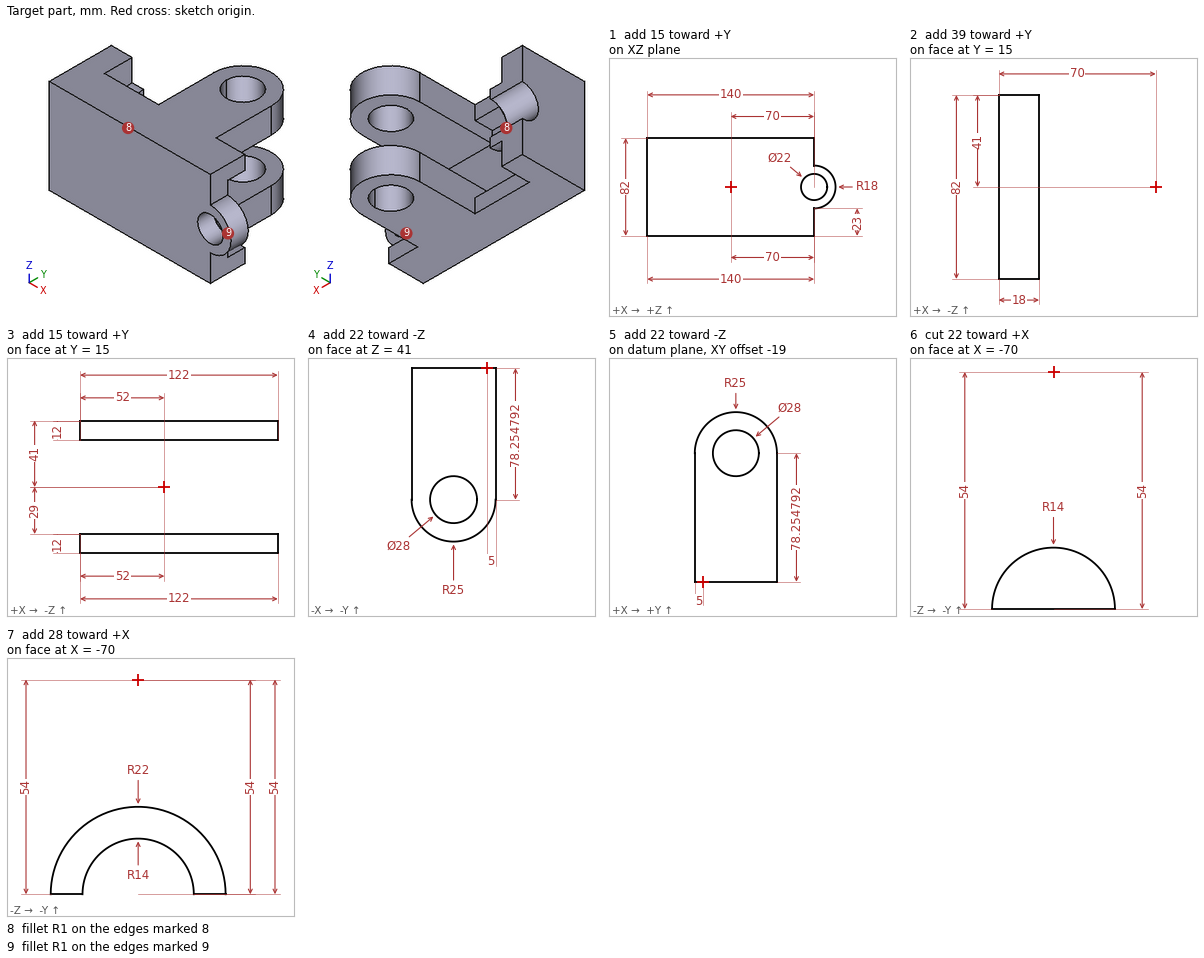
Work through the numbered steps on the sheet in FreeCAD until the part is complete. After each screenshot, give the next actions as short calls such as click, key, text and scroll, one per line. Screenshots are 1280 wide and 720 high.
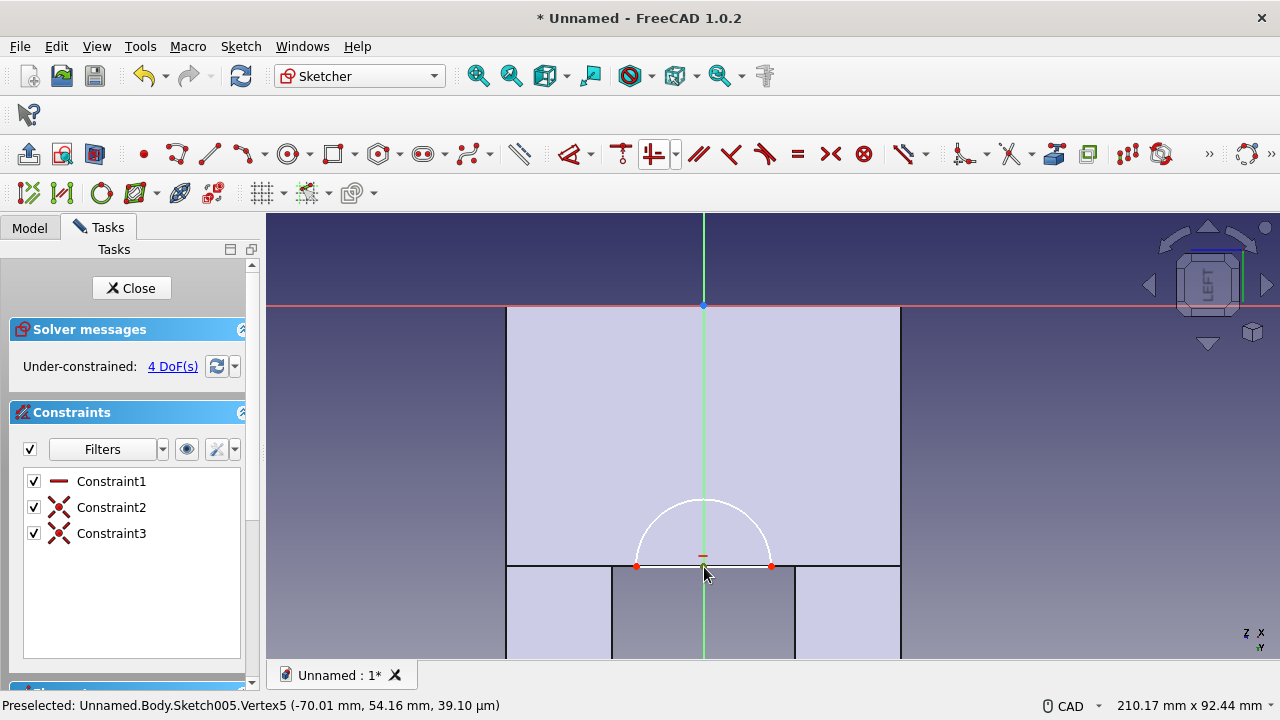
click(704, 603)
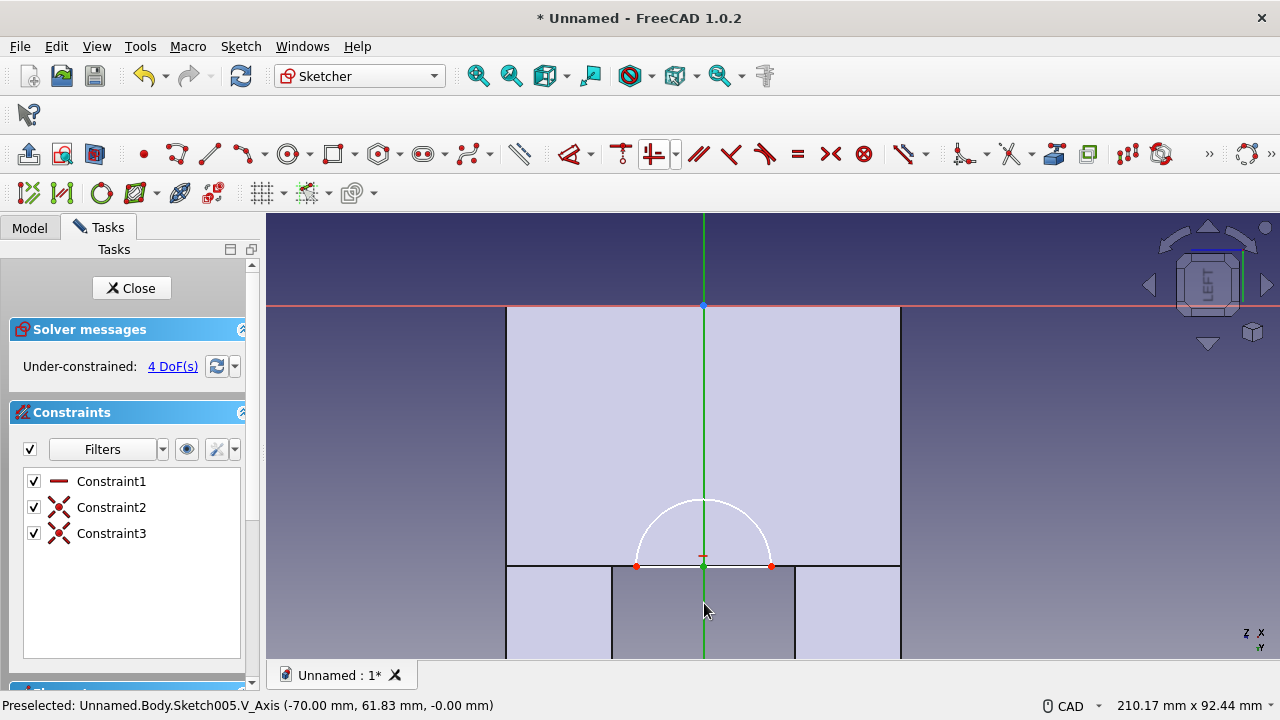
click(621, 154)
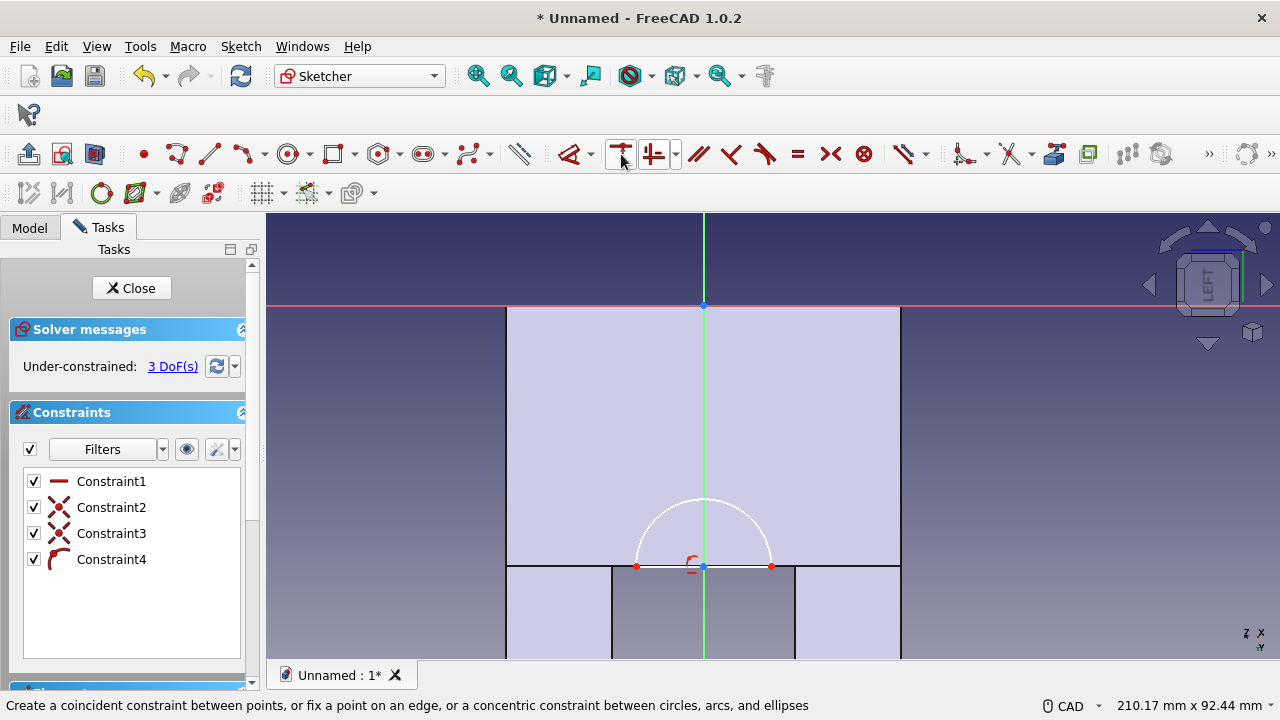
click(568, 154)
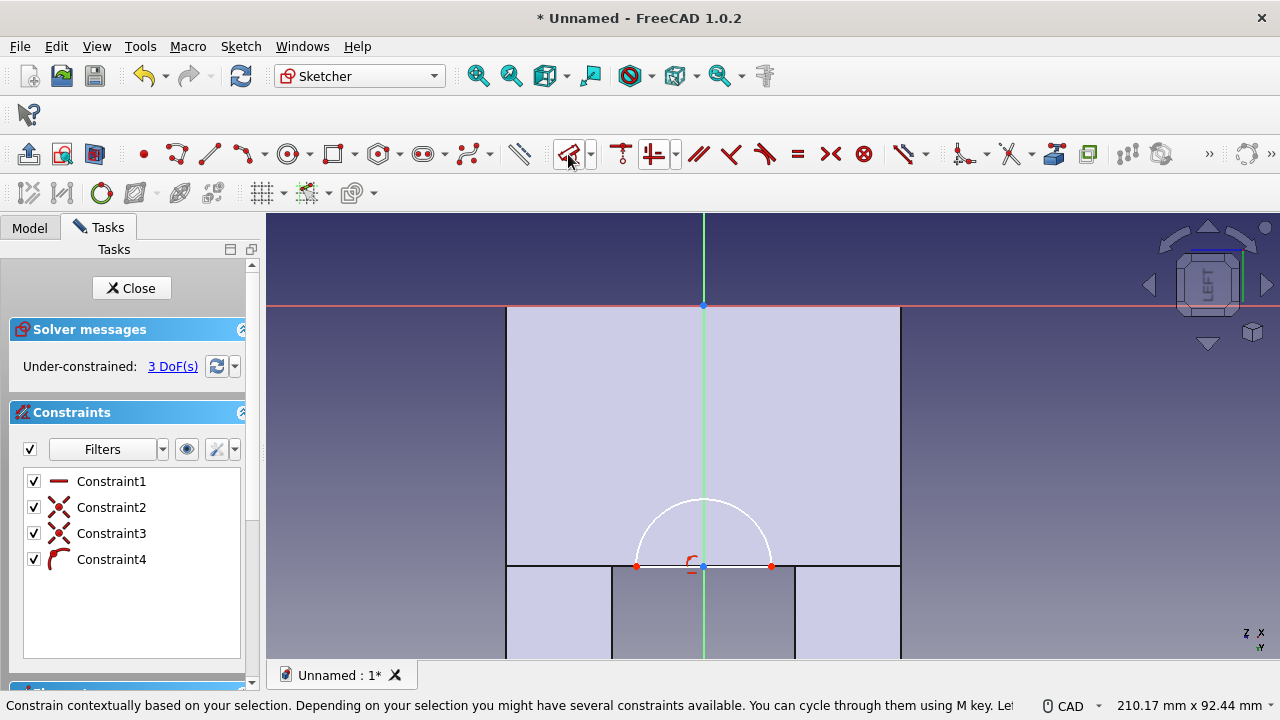
click(743, 512)
click(762, 486)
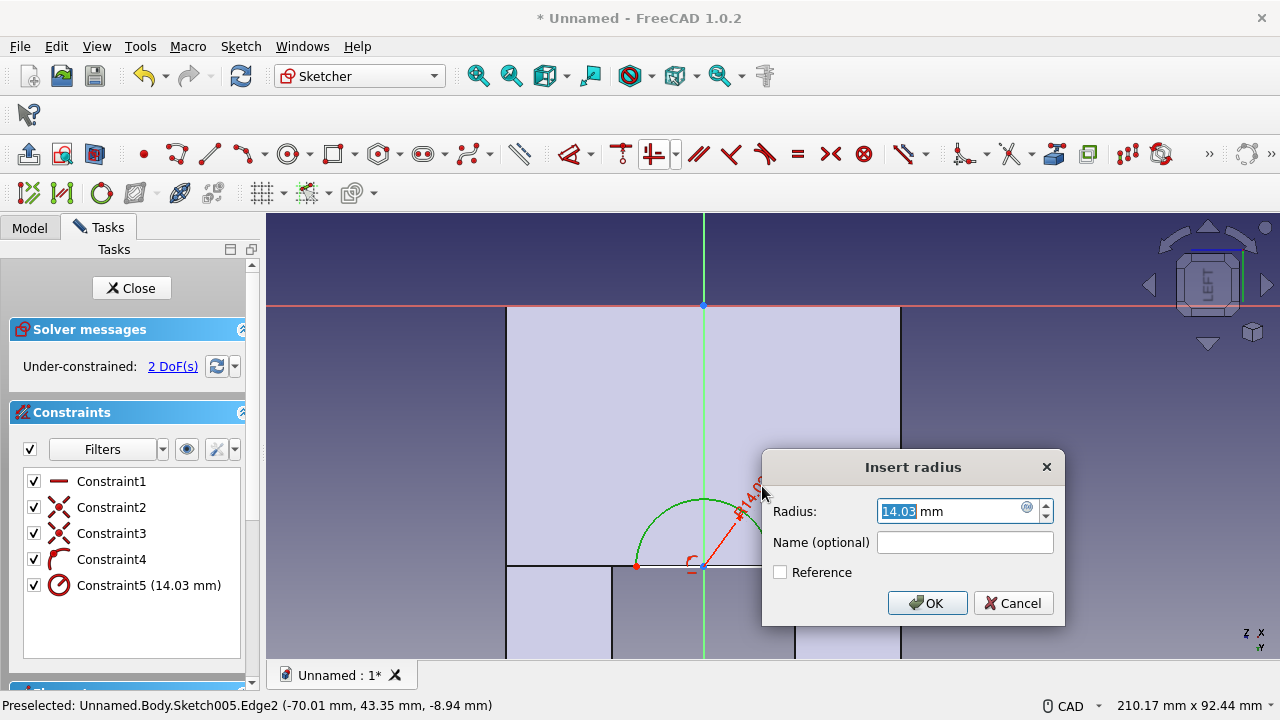
text(14)
key(Return)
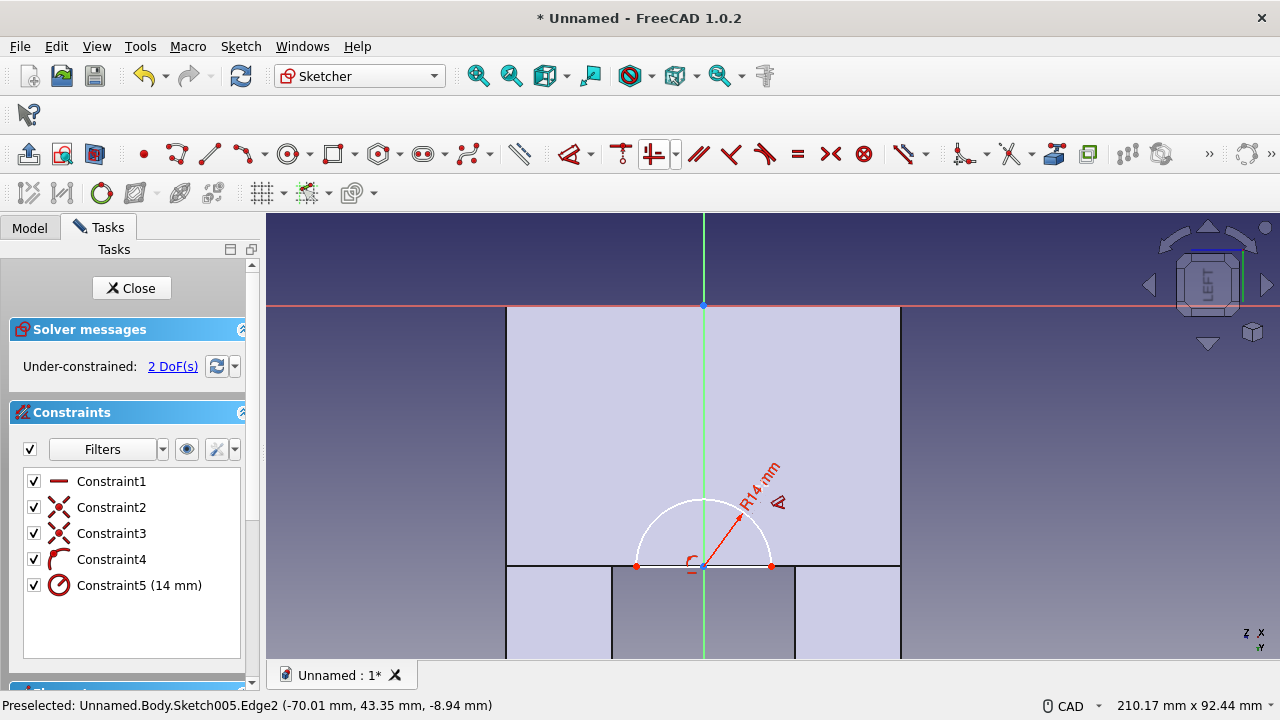
click(636, 567)
click(602, 436)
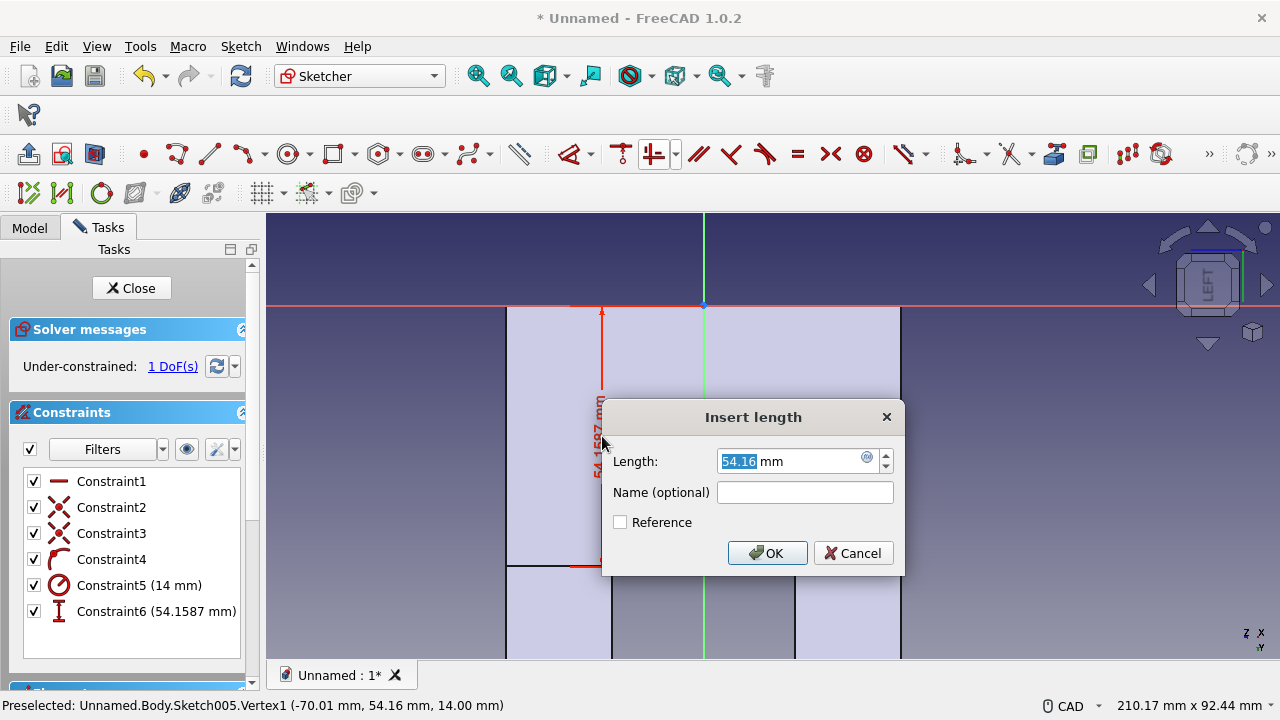
text(54)
key(Return)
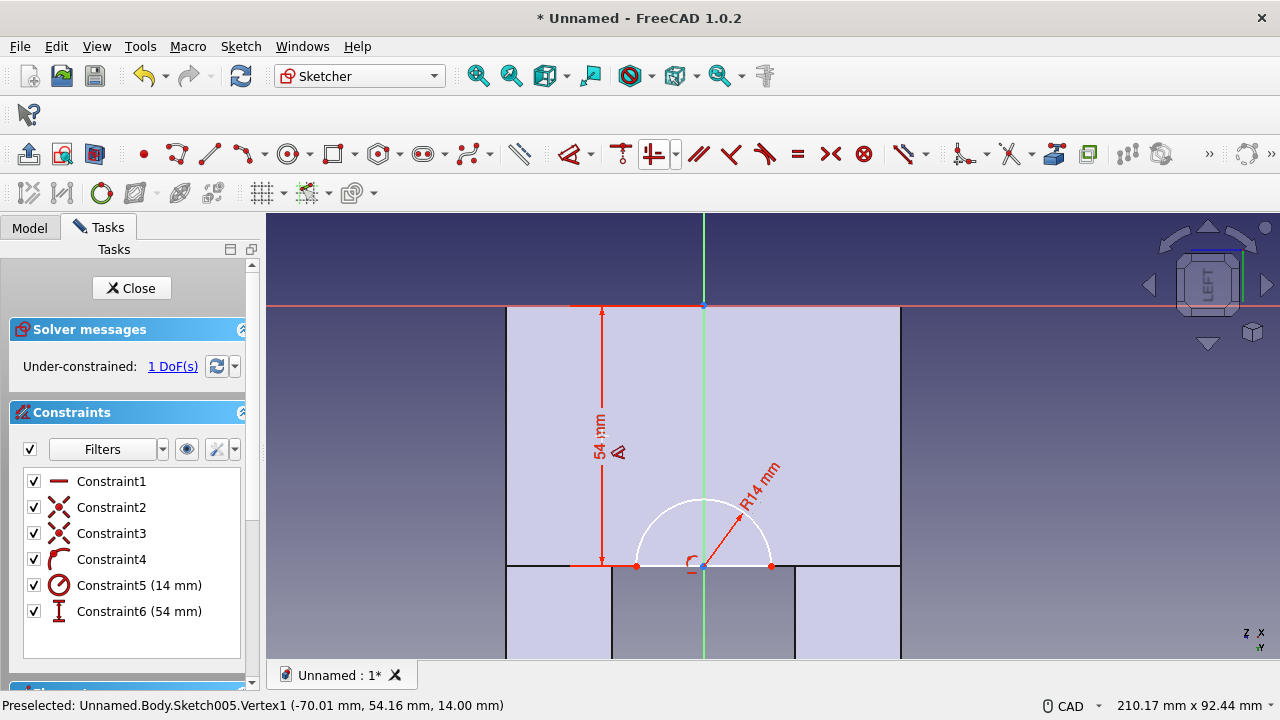
click(704, 567)
click(738, 436)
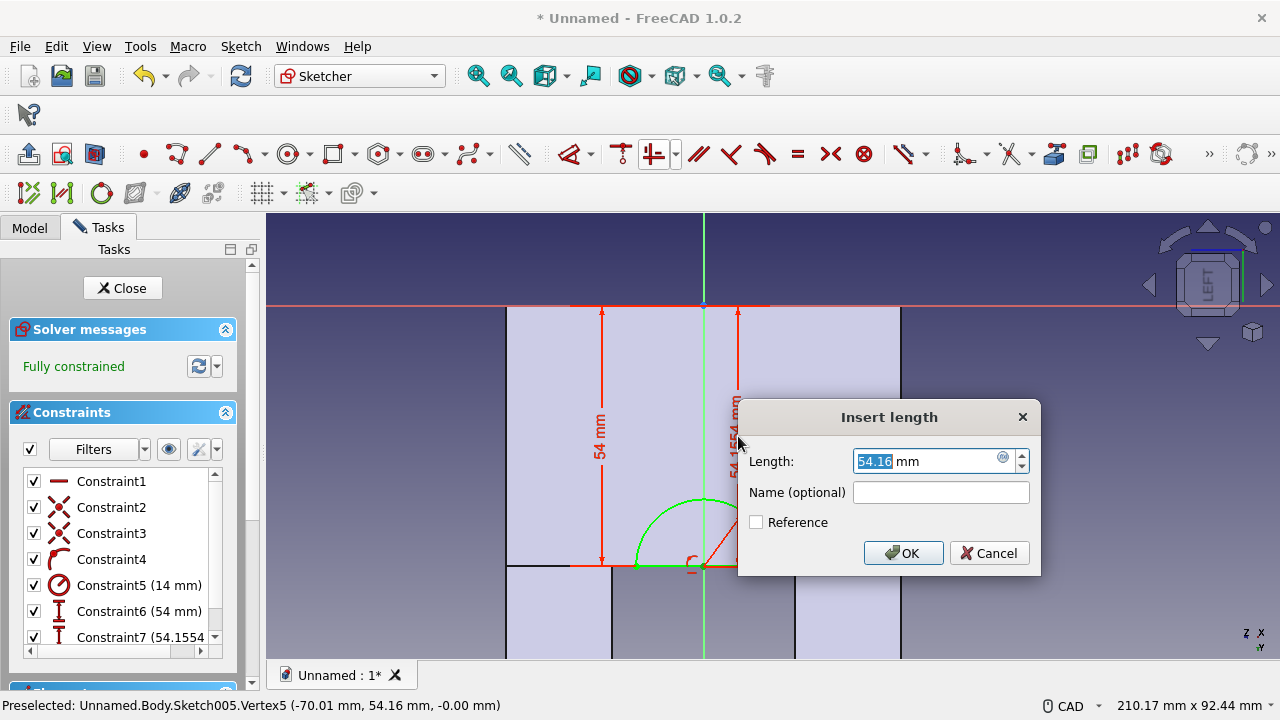
text(54)
key(Return)
key(Escape)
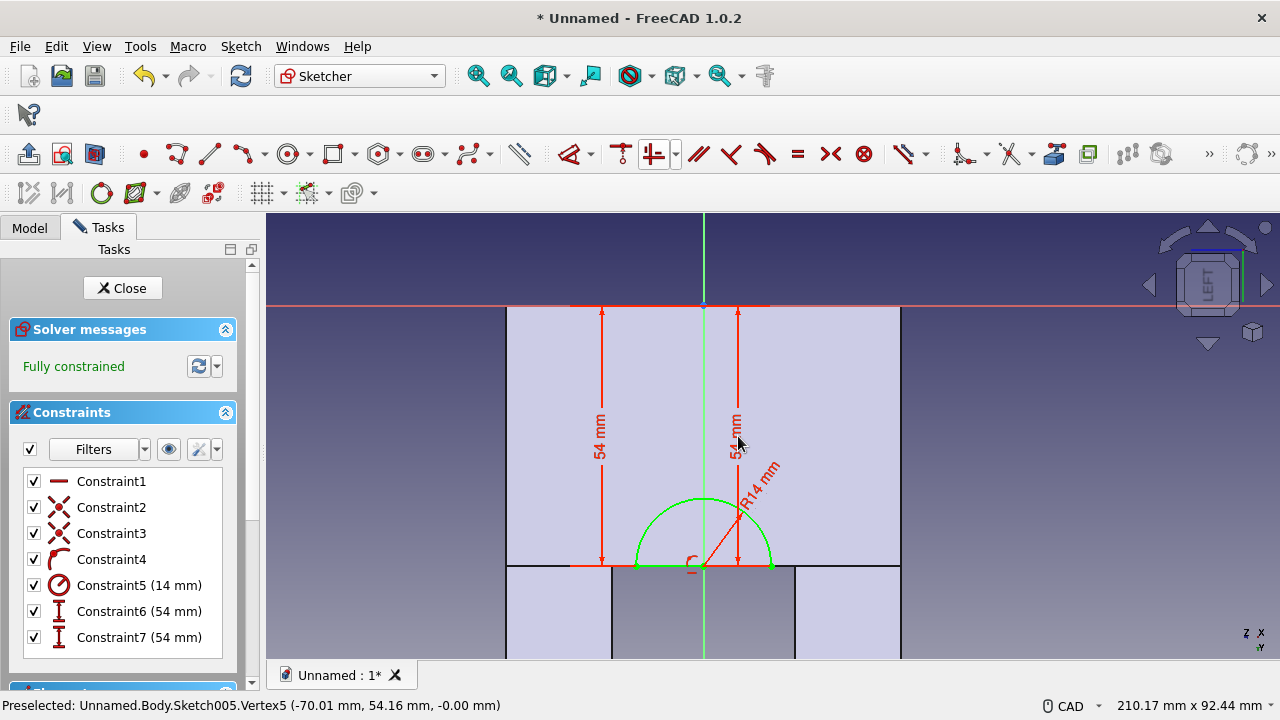
click(123, 288)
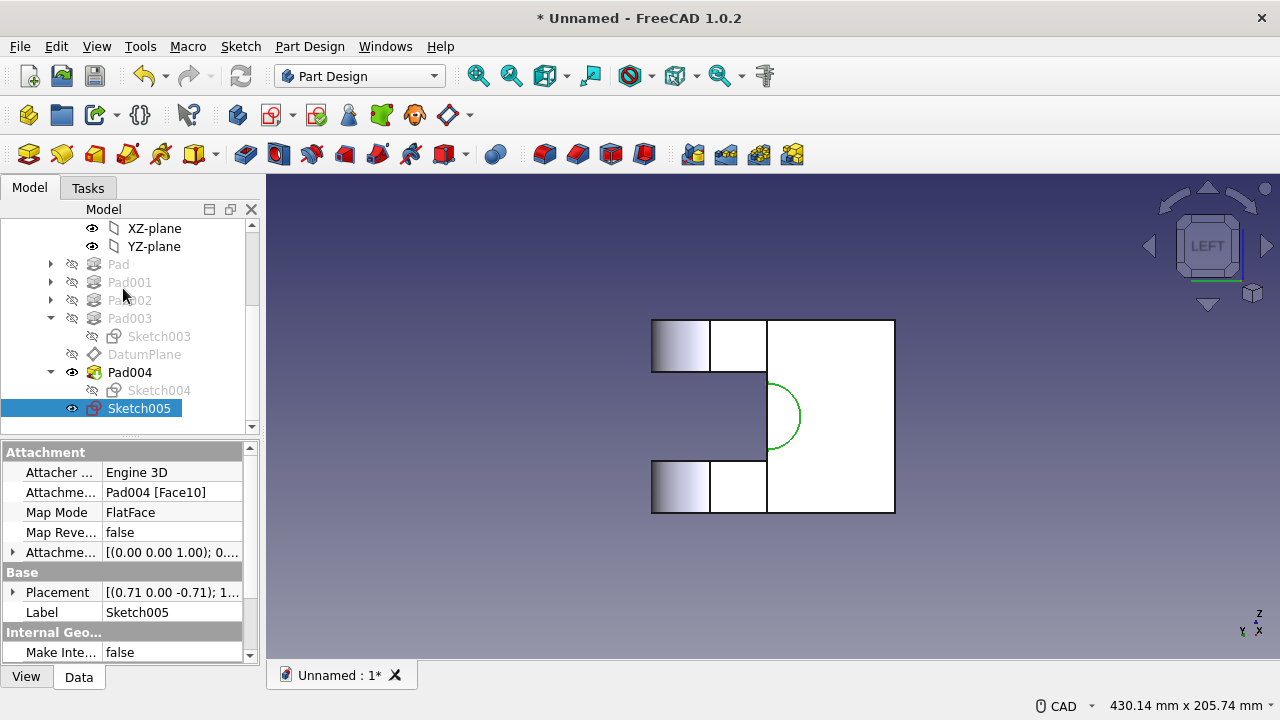
click(246, 154)